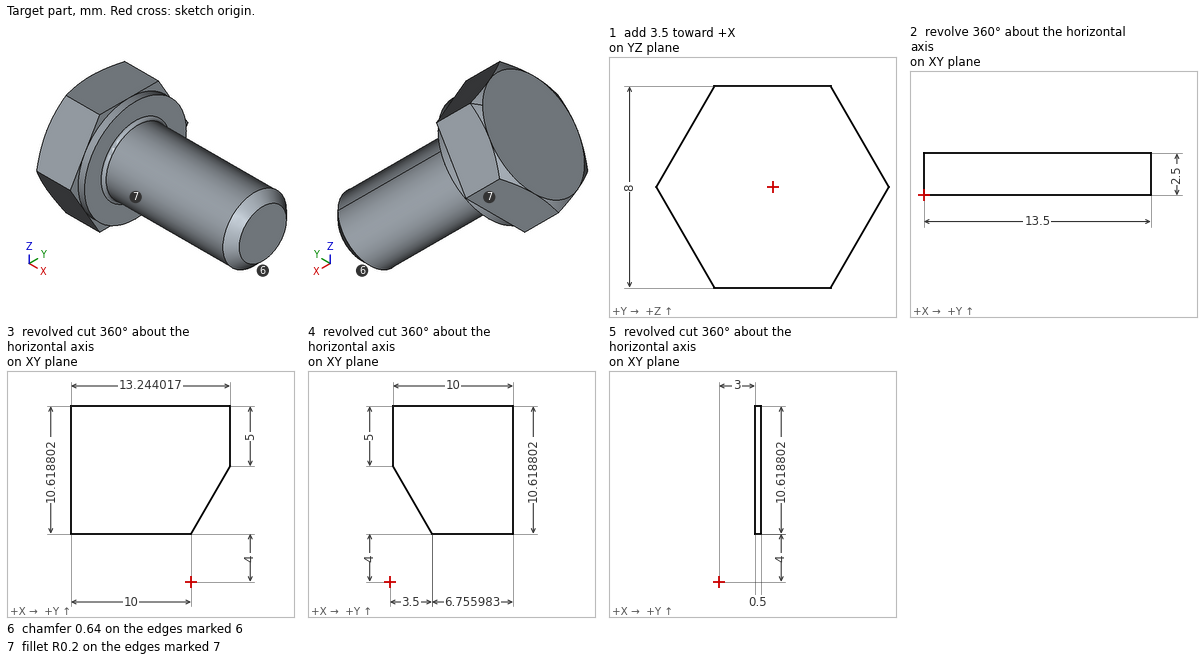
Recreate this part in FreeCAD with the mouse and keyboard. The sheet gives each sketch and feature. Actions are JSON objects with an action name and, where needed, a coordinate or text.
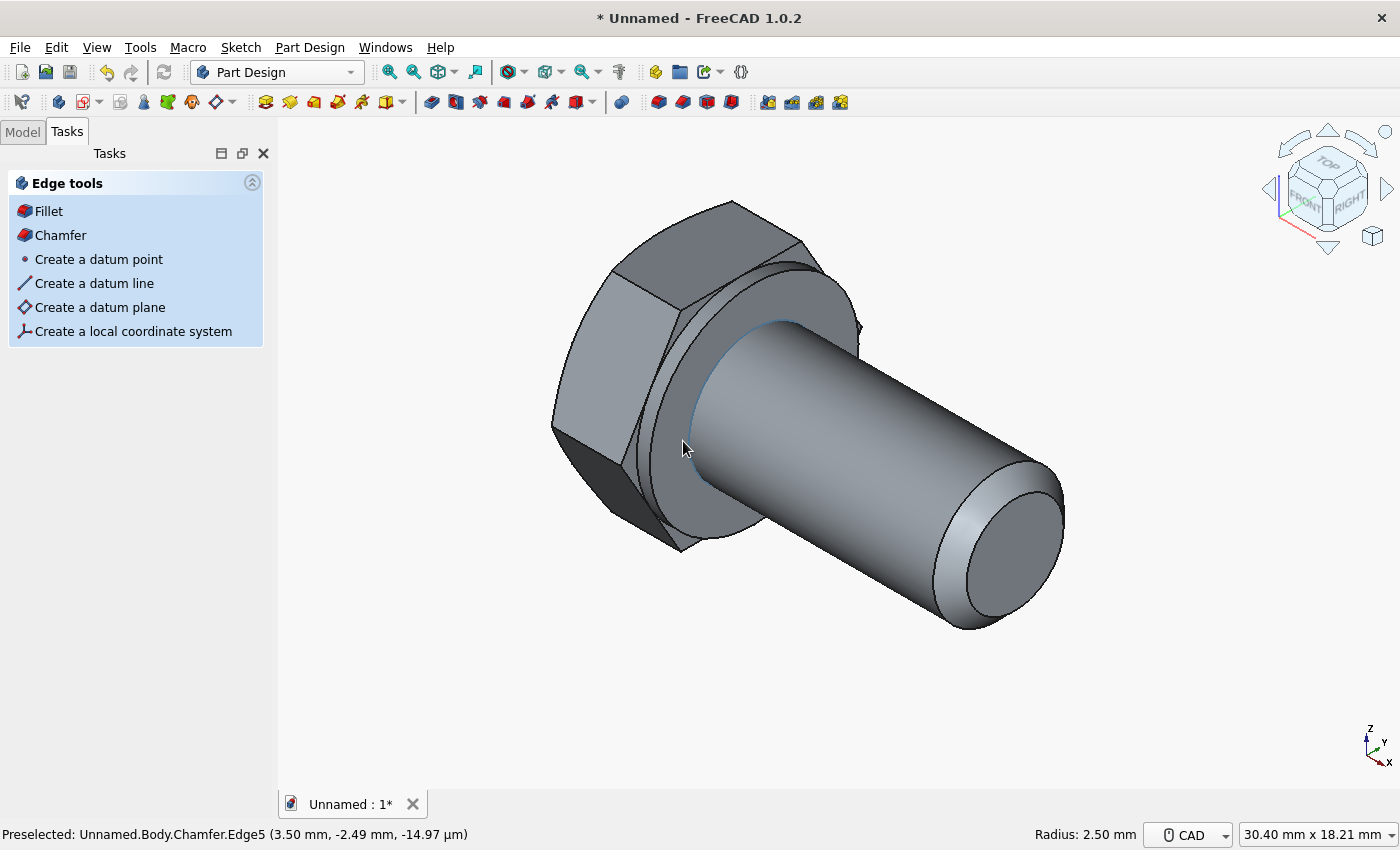
{"action": "left_click", "coordinate": [660, 102]}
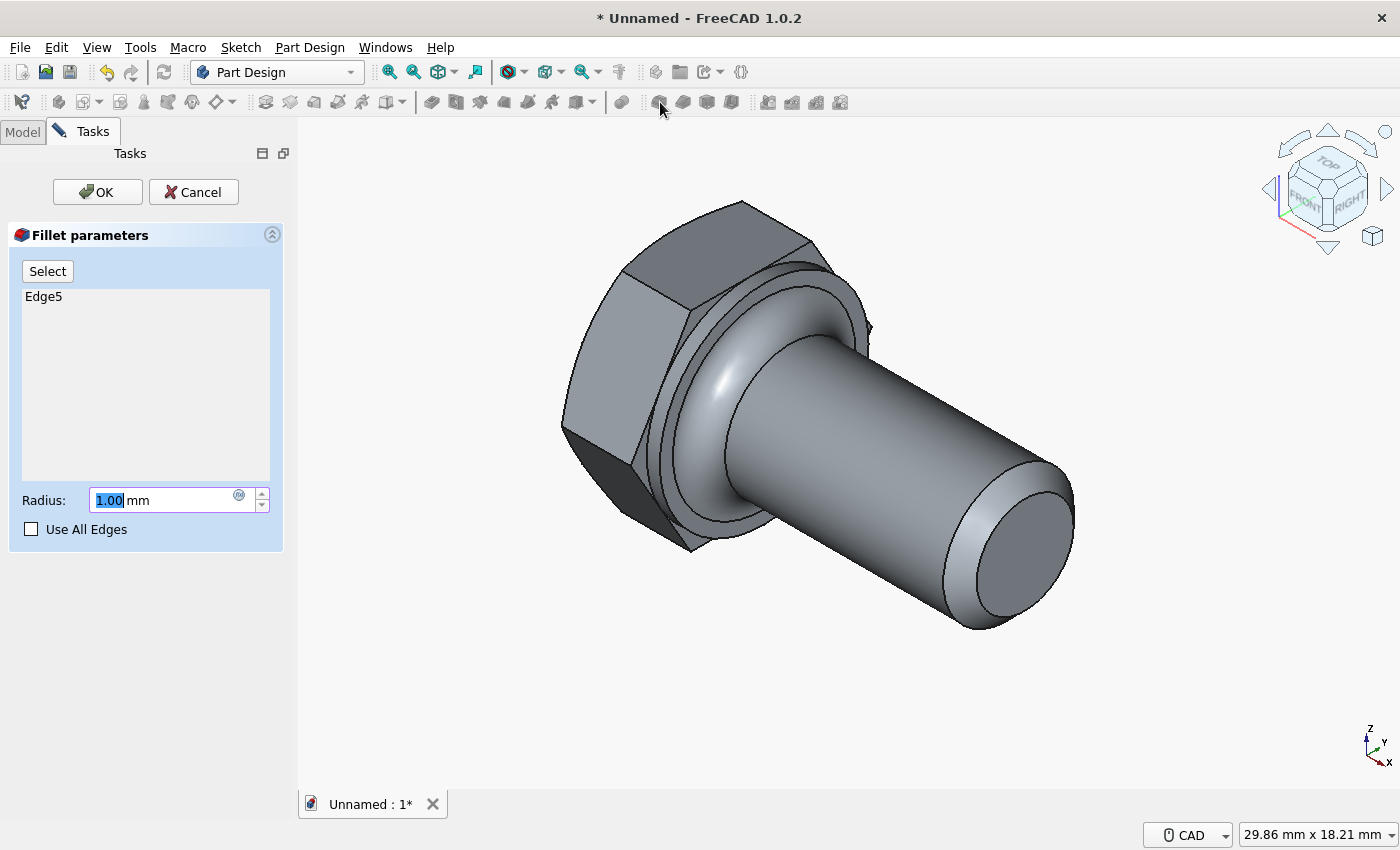
{"action": "type", "text": "0.2"}
{"action": "key", "text": "Tab"}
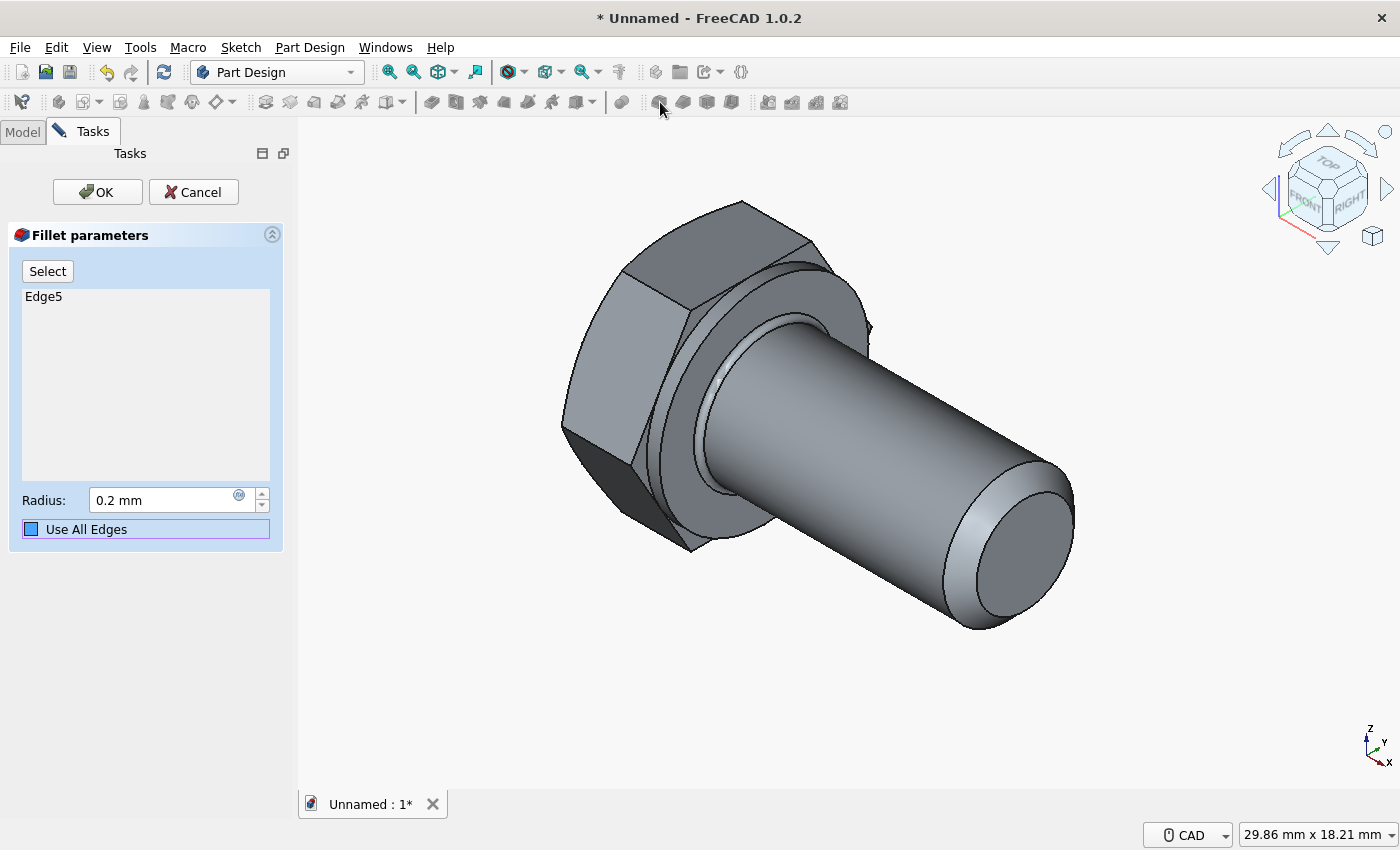
{"action": "left_click", "coordinate": [98, 192]}